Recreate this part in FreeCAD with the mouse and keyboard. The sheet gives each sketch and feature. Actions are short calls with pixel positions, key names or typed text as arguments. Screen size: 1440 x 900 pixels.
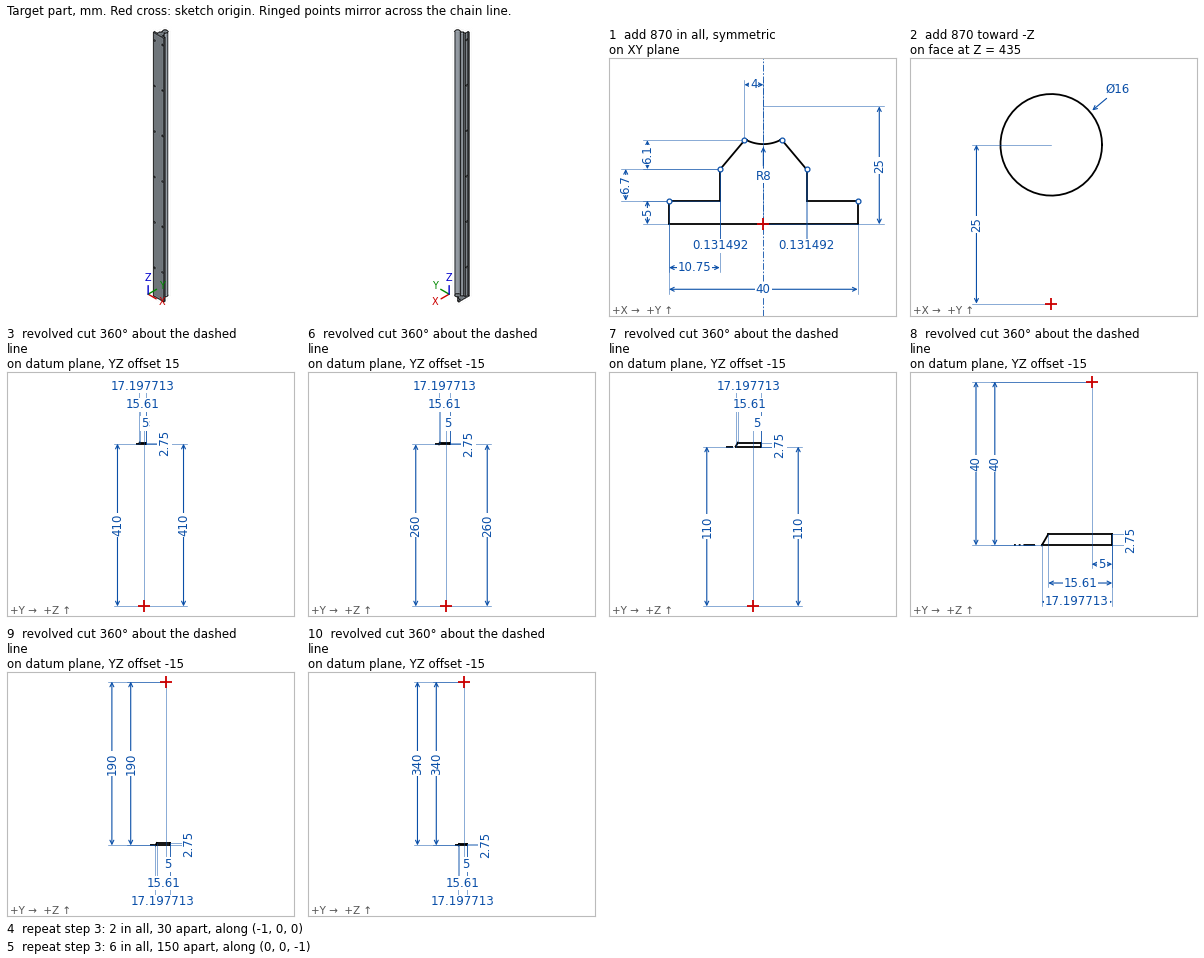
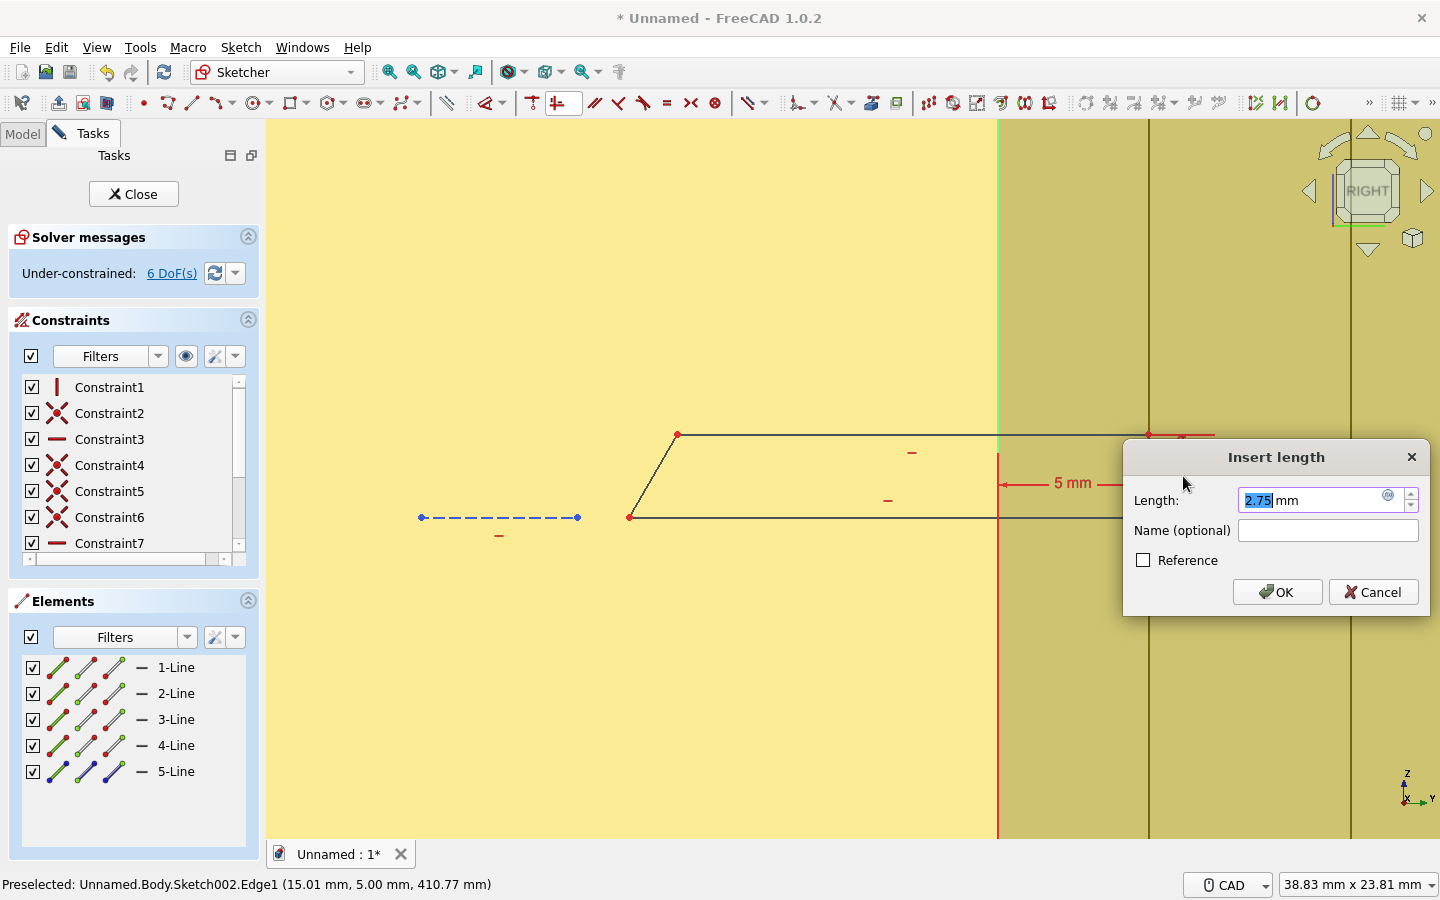
text(2.75)
key(Return)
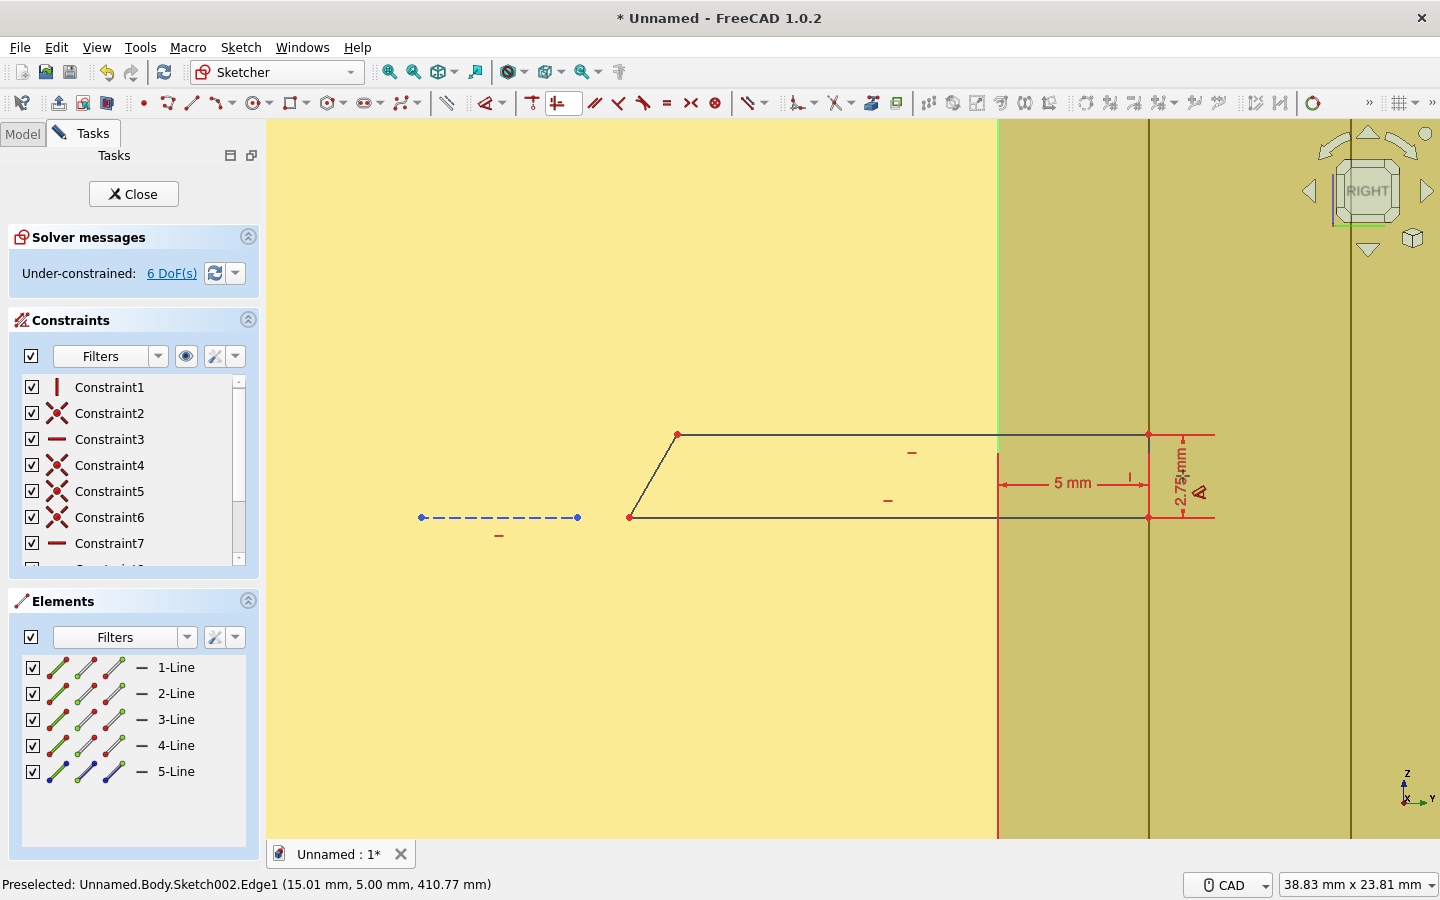
click(1149, 518)
click(1183, 665)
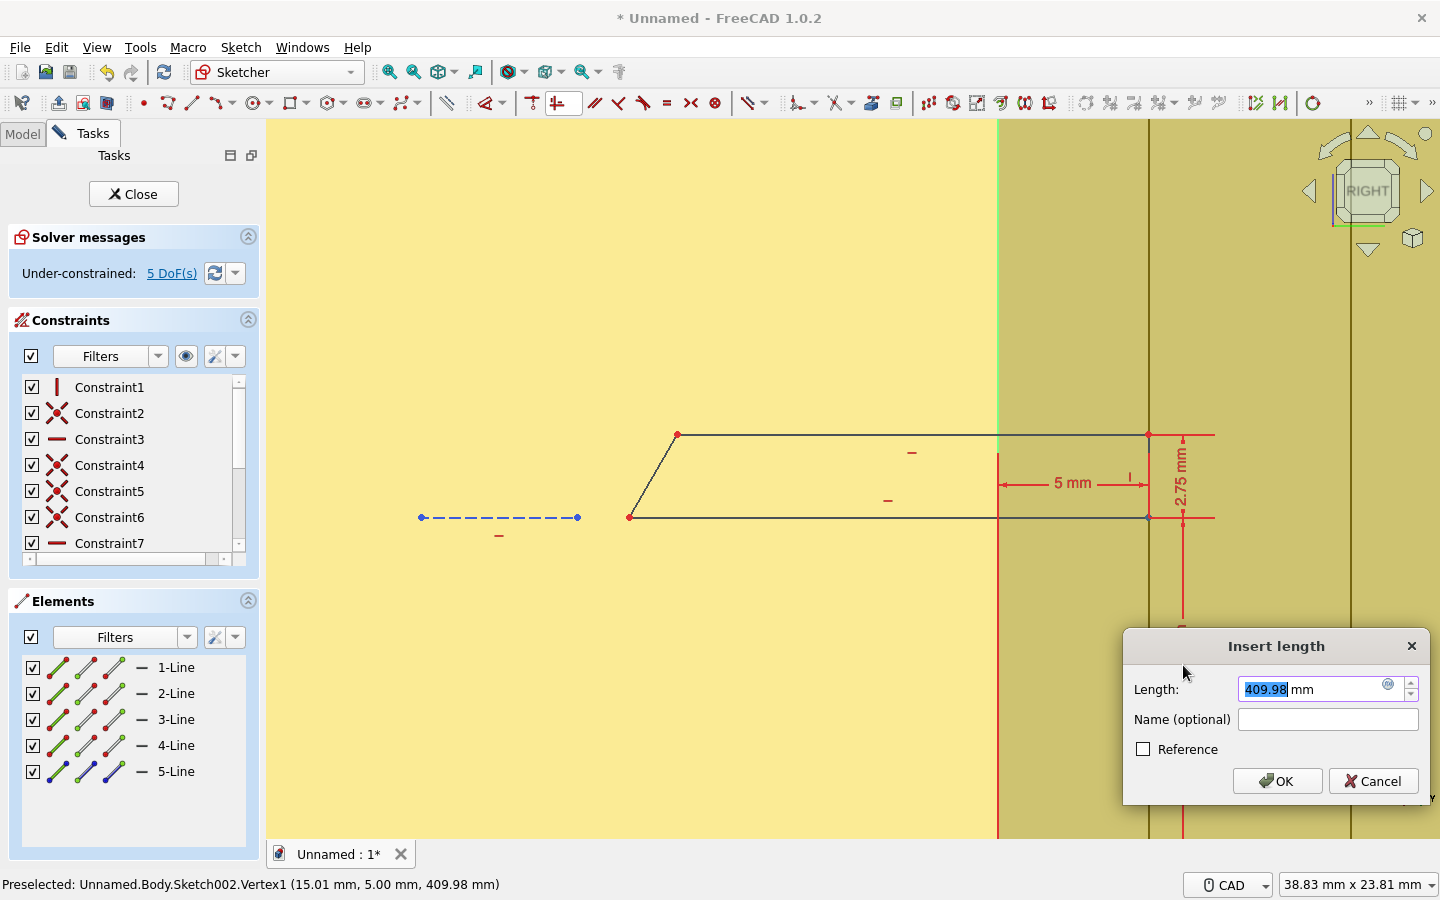
text(410)
key(Return)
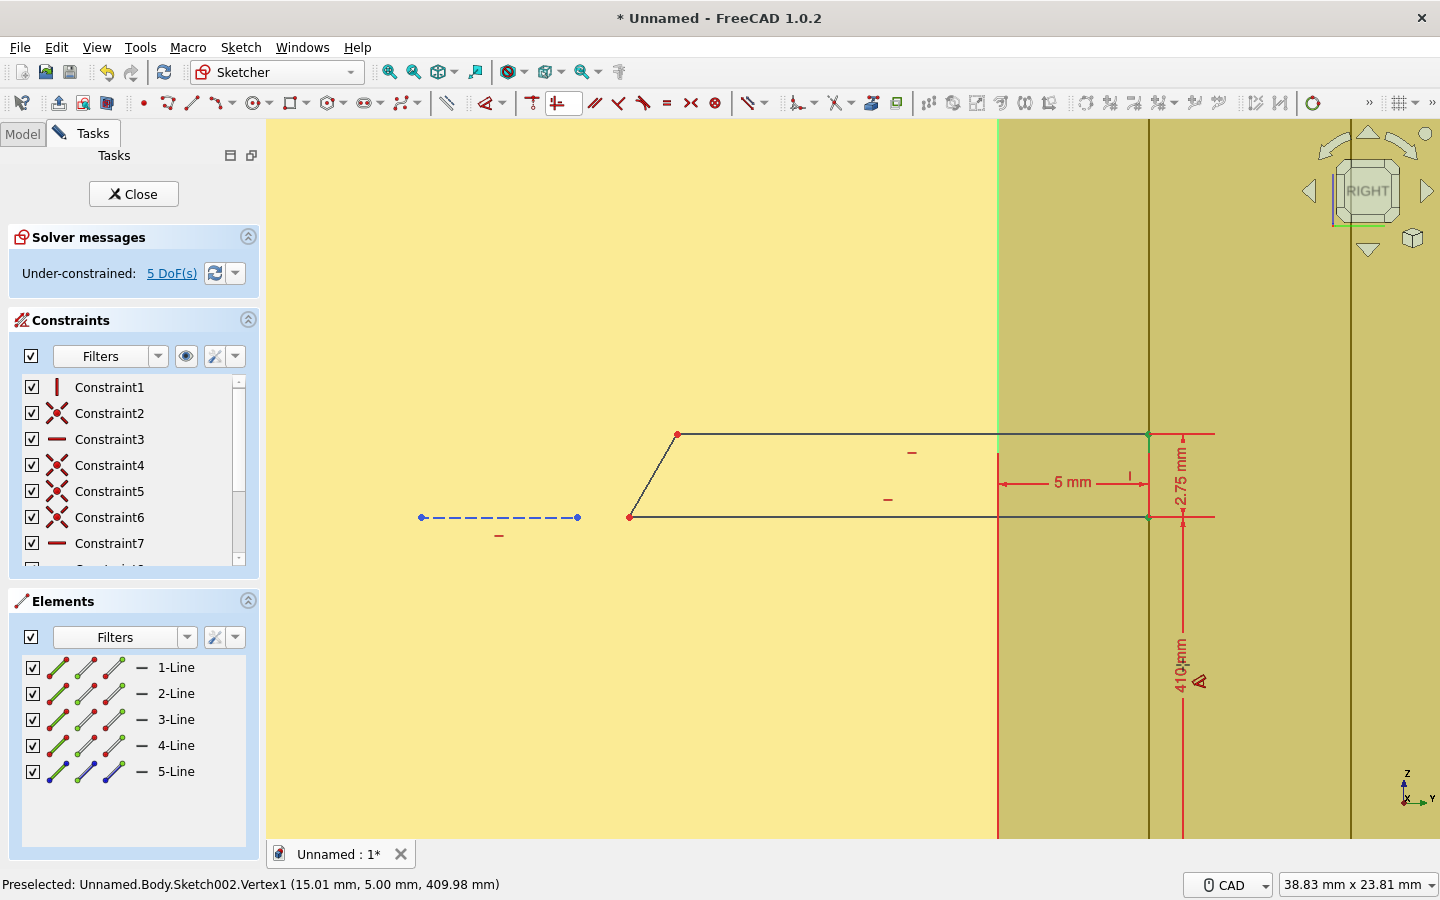
click(577, 518)
click(1032, 665)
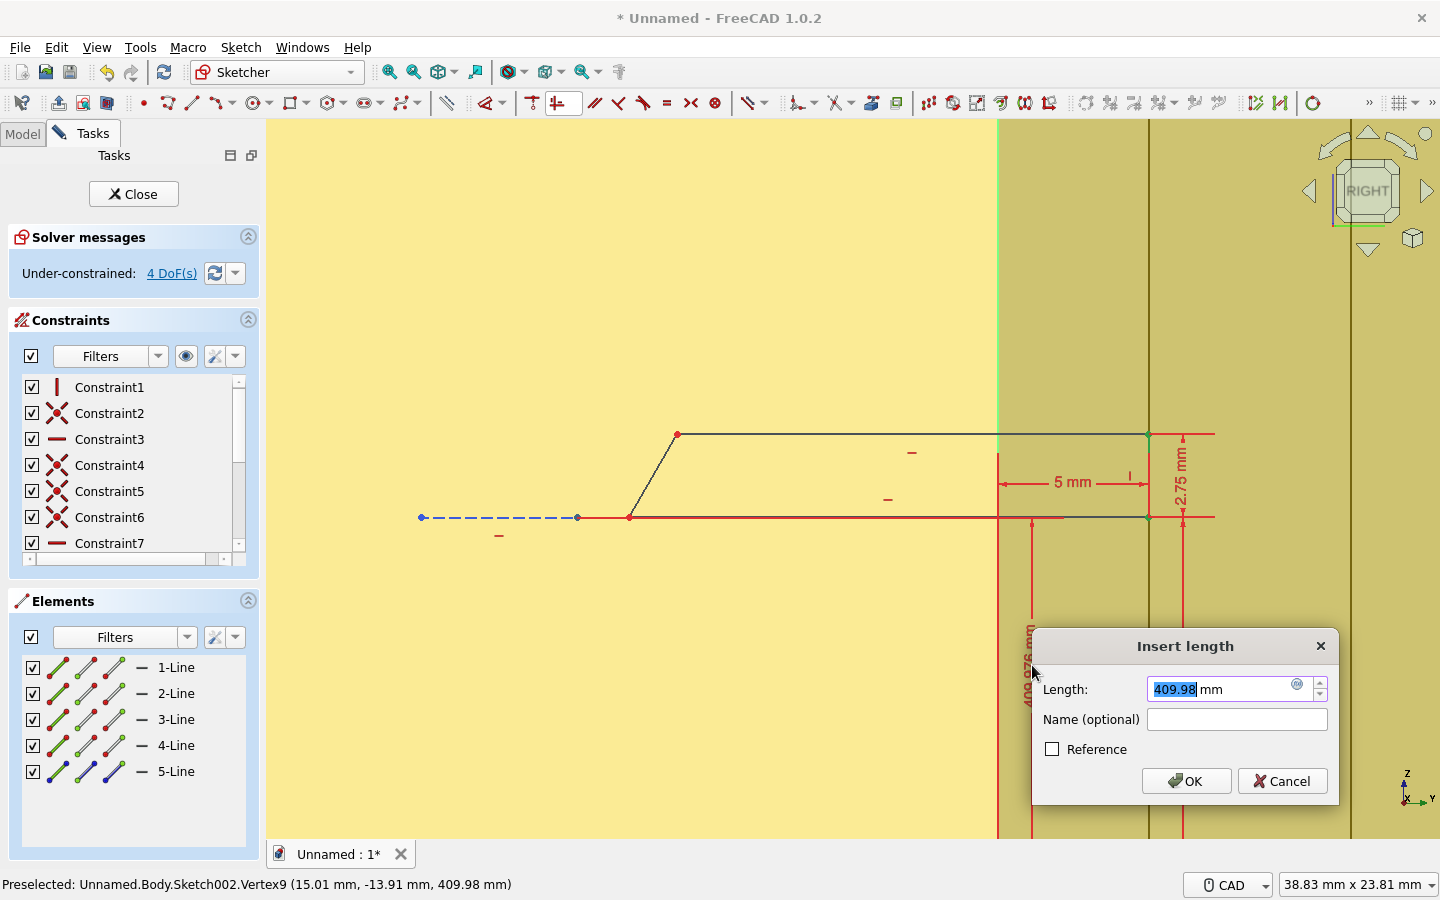
text(410)
key(Return)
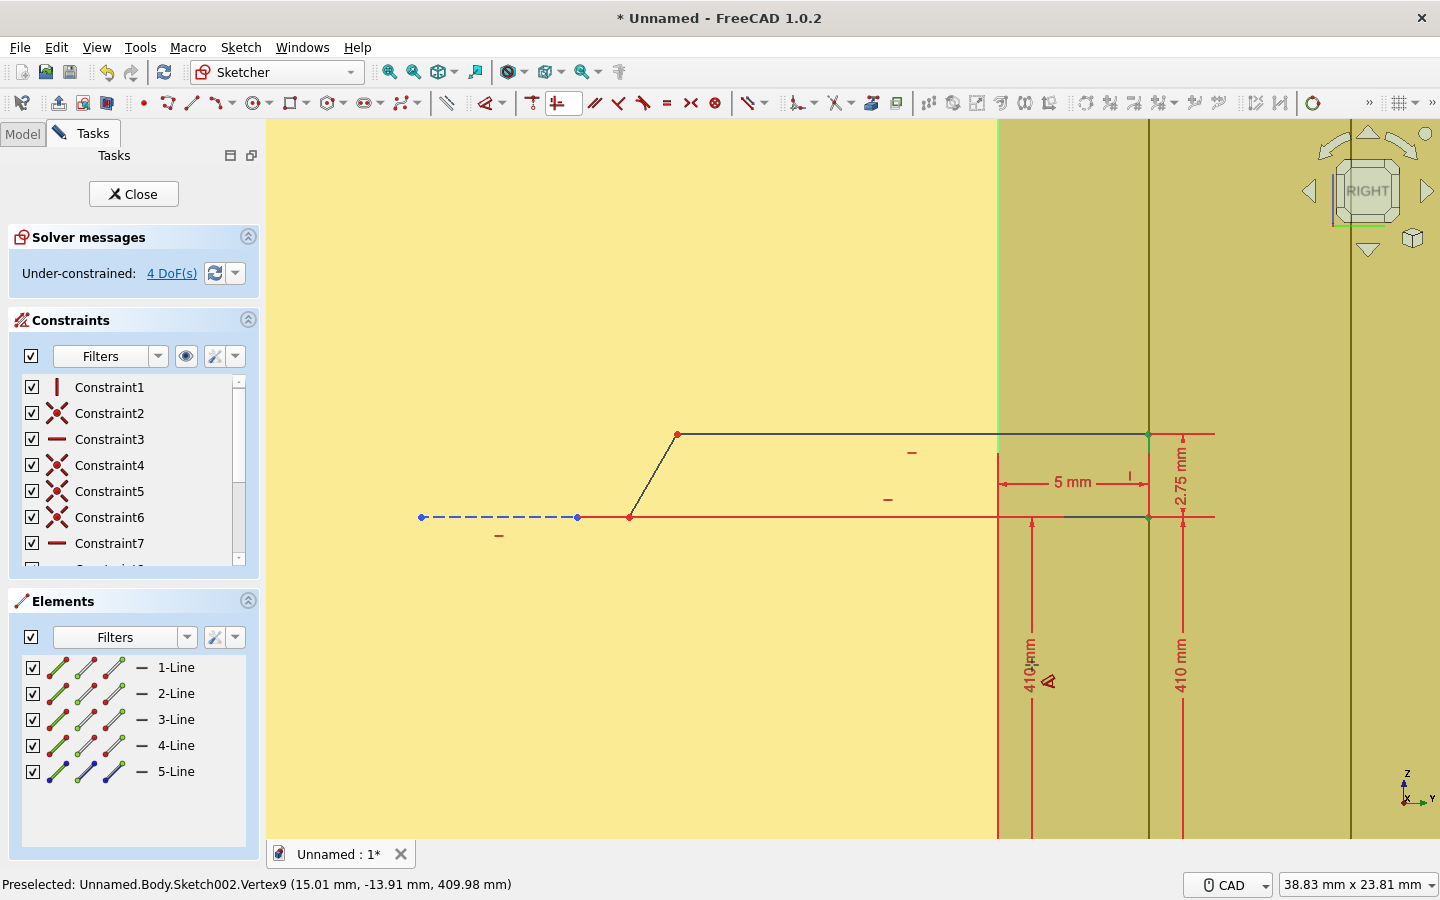
scroll(1007, 434, up, 2)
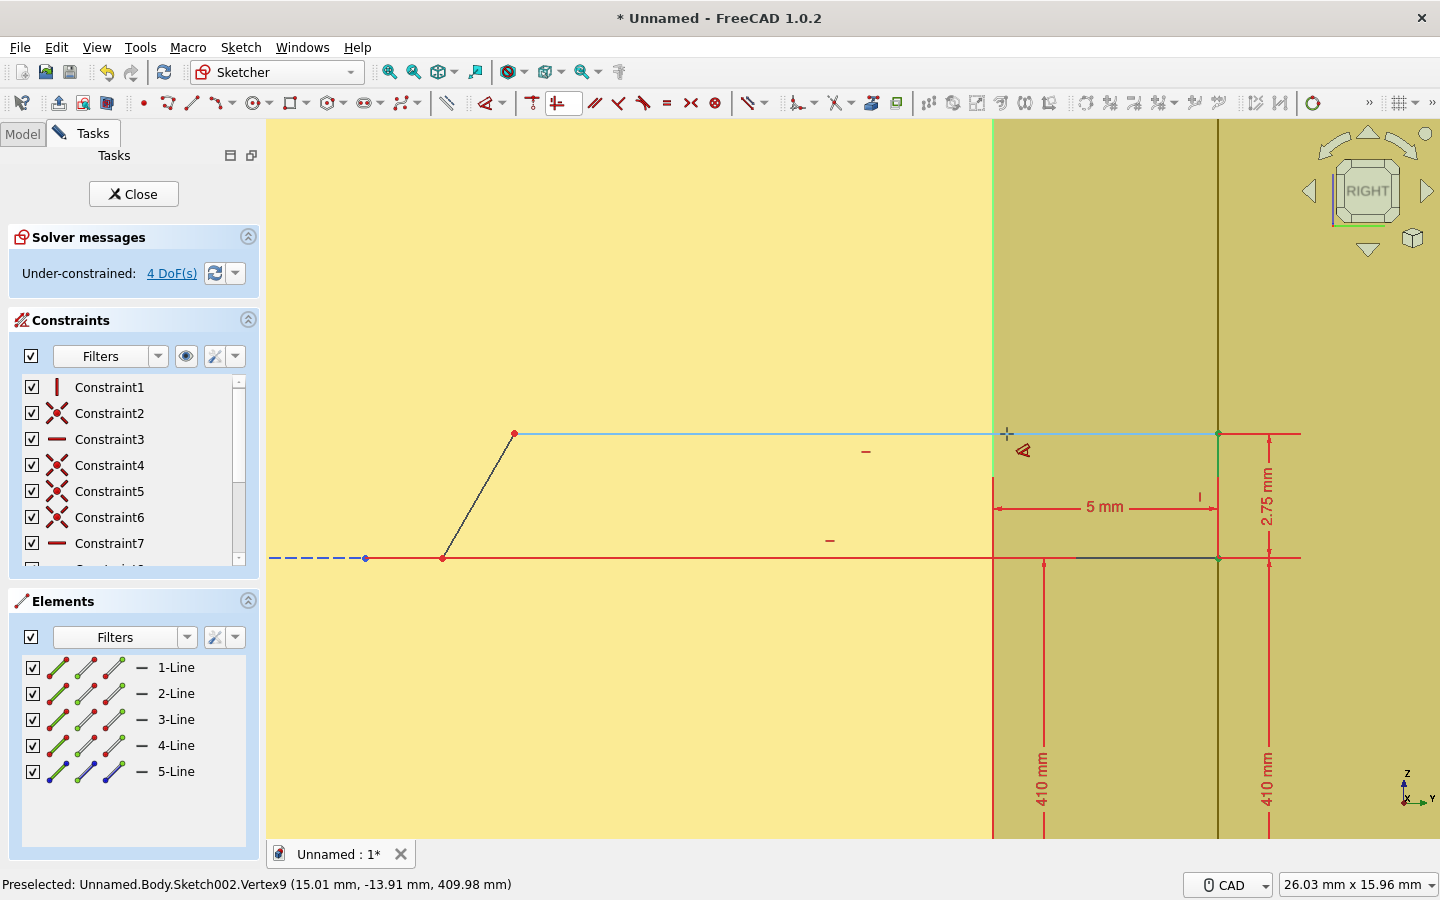
click(1007, 434)
click(866, 400)